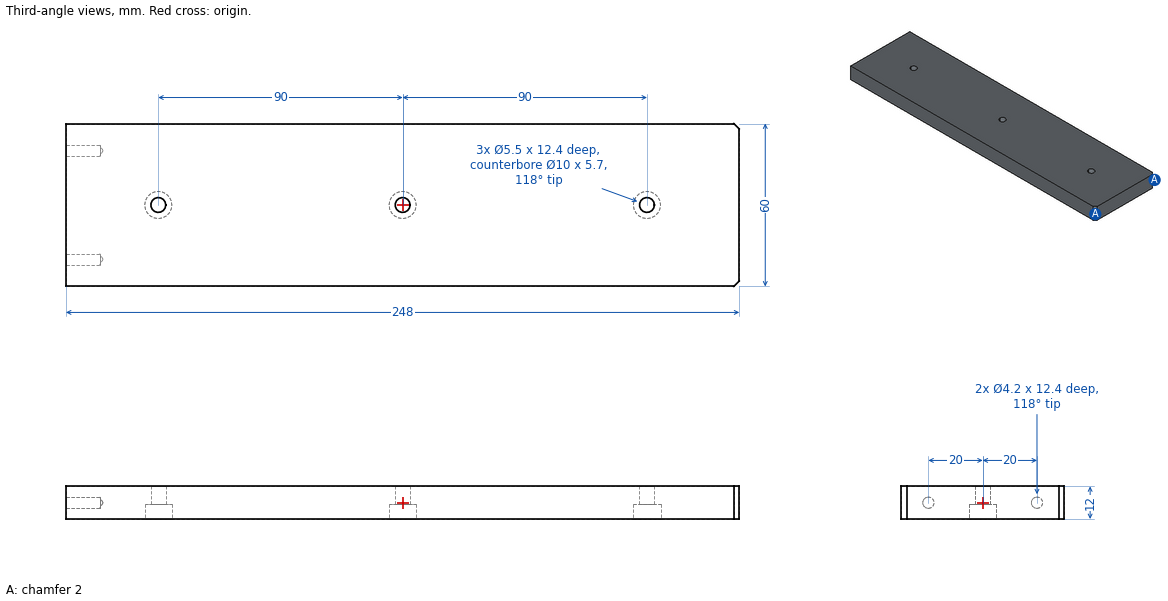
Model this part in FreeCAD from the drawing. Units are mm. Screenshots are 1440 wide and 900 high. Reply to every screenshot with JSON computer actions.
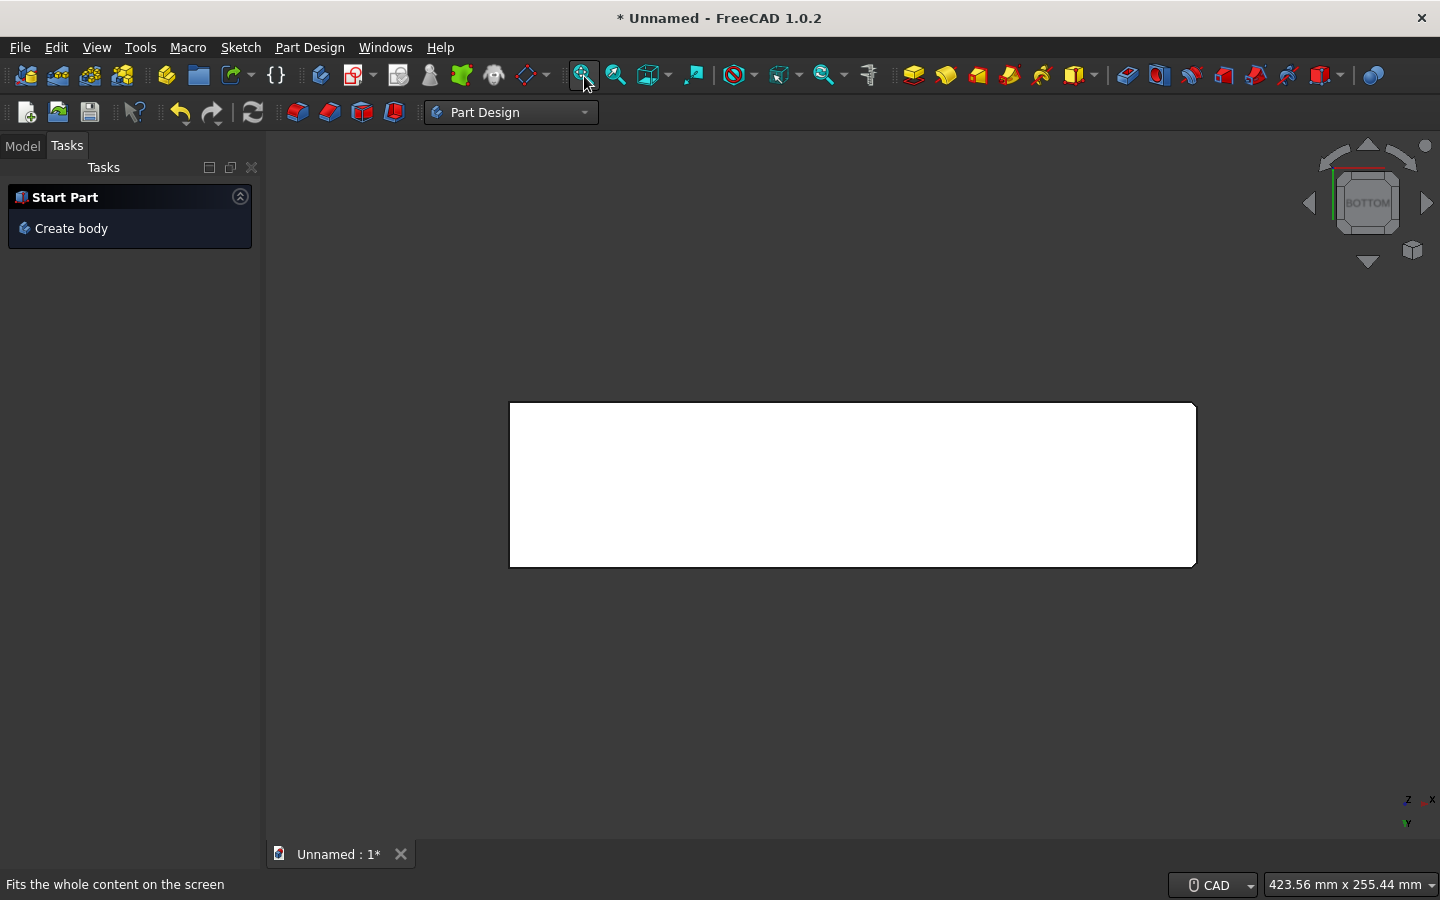
{"action": "left_click", "coordinate": [1049, 484]}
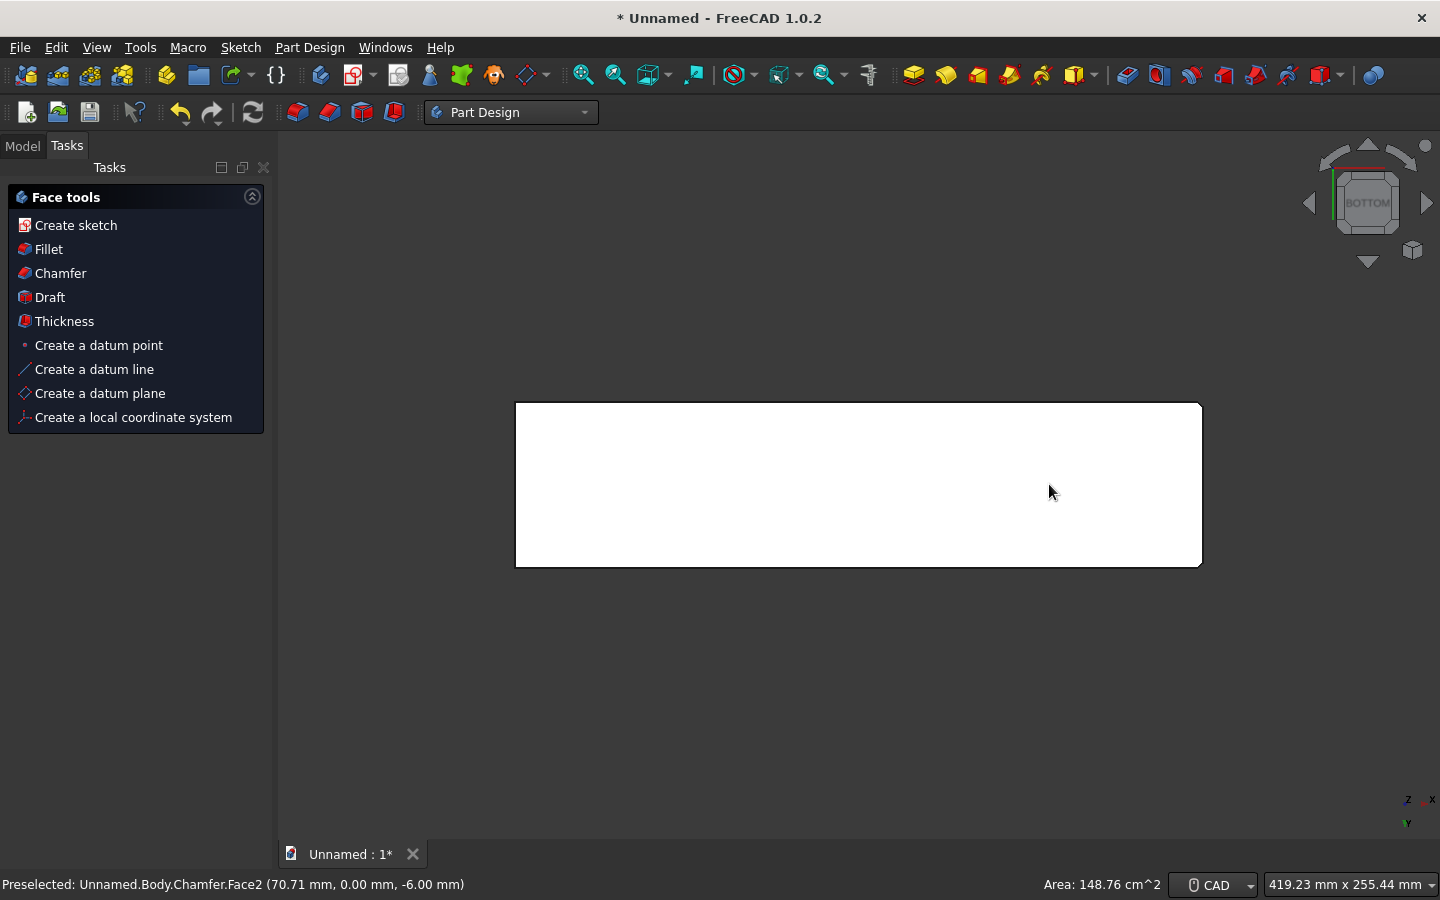
{"action": "left_click", "coordinate": [354, 76]}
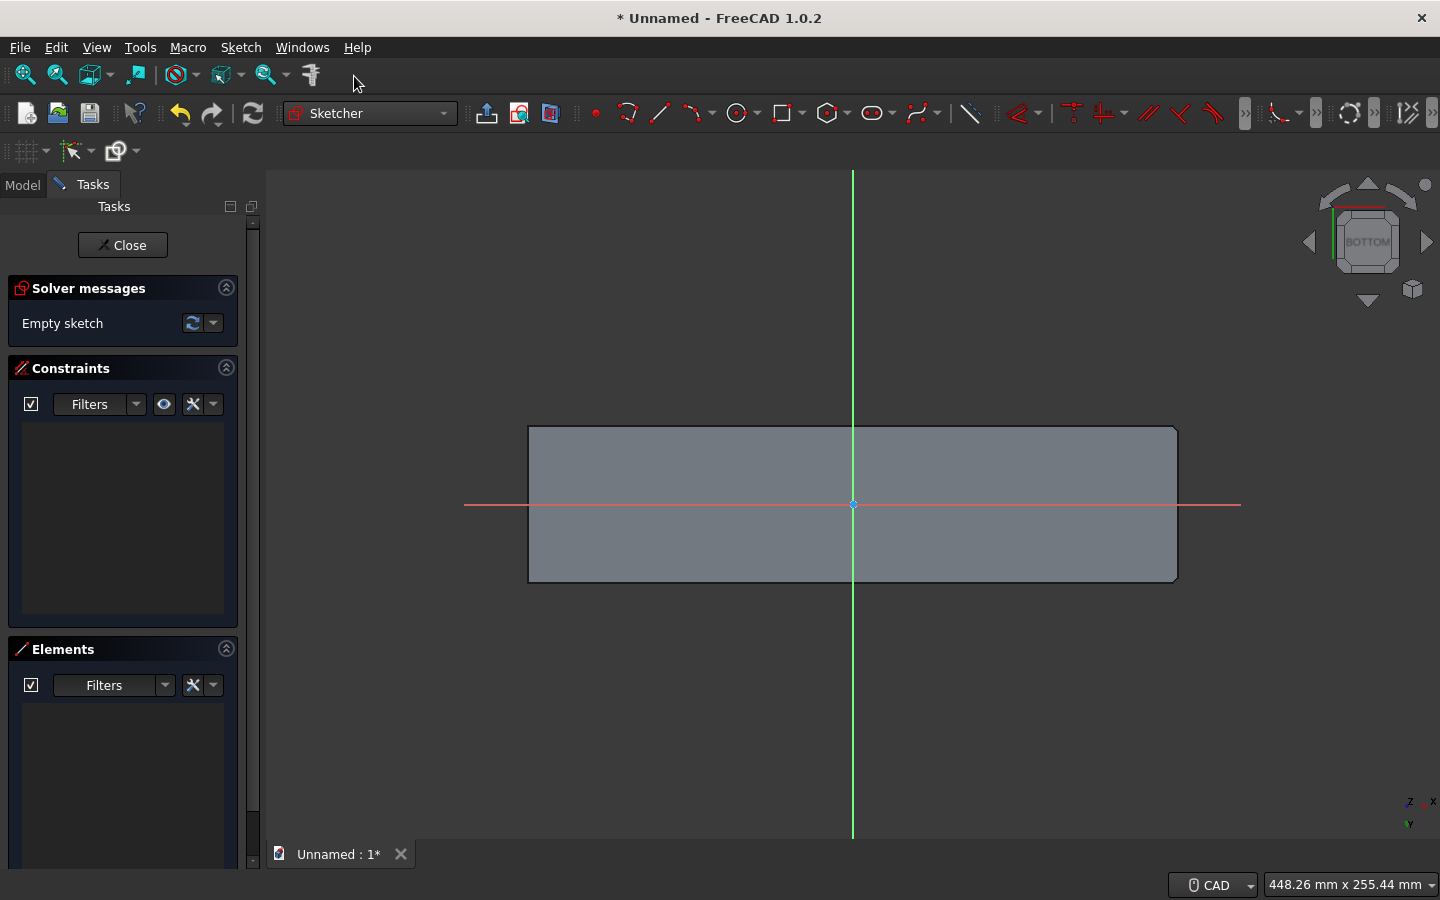
{"action": "scroll", "coordinate": [992, 504], "scroll_direction": "up", "scroll_amount": 2}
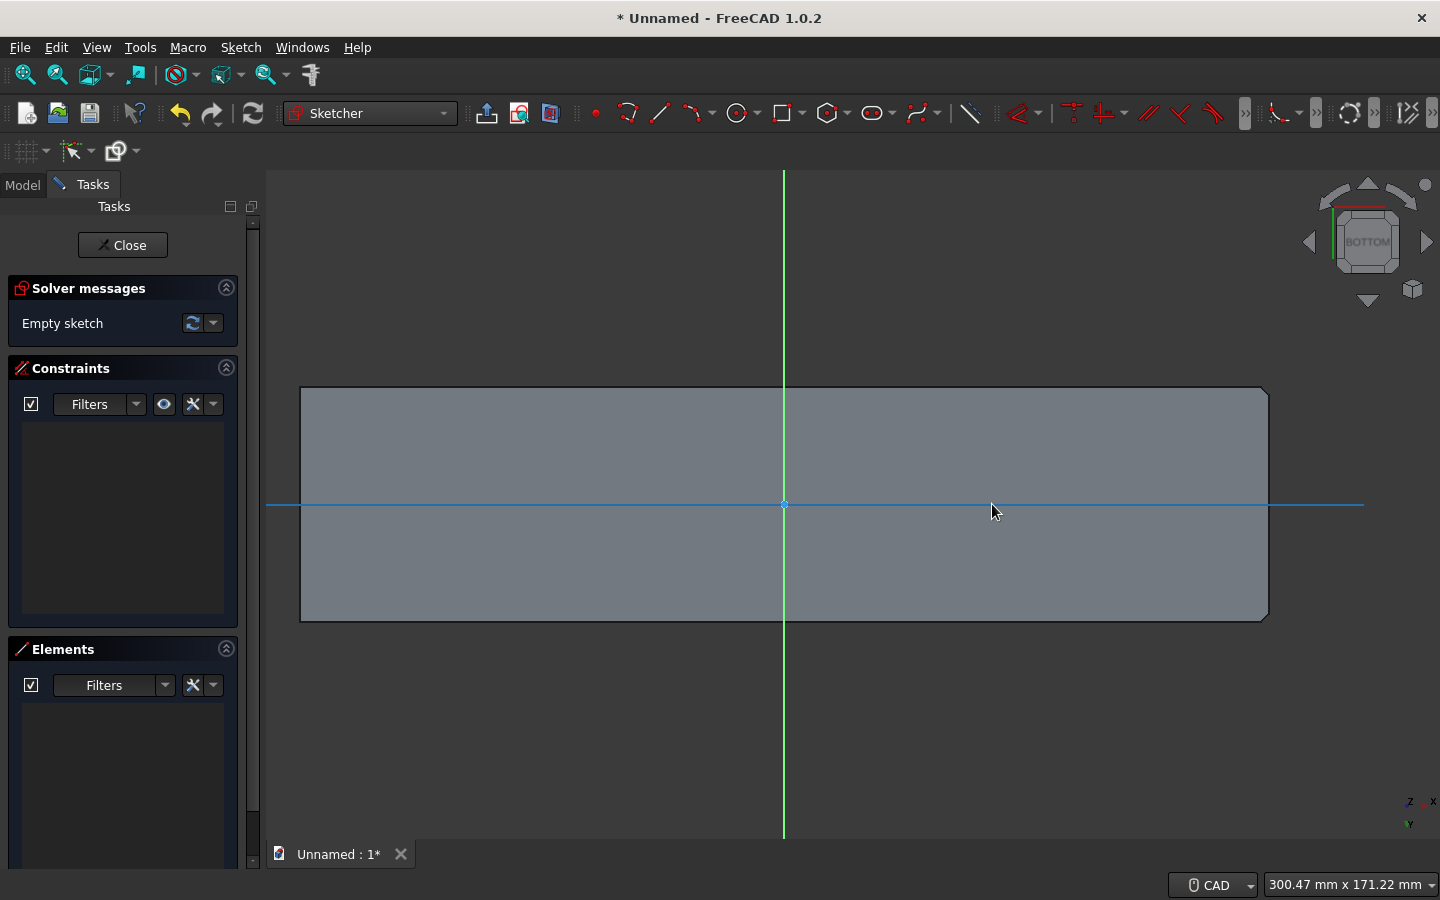
{"action": "left_click", "coordinate": [738, 114]}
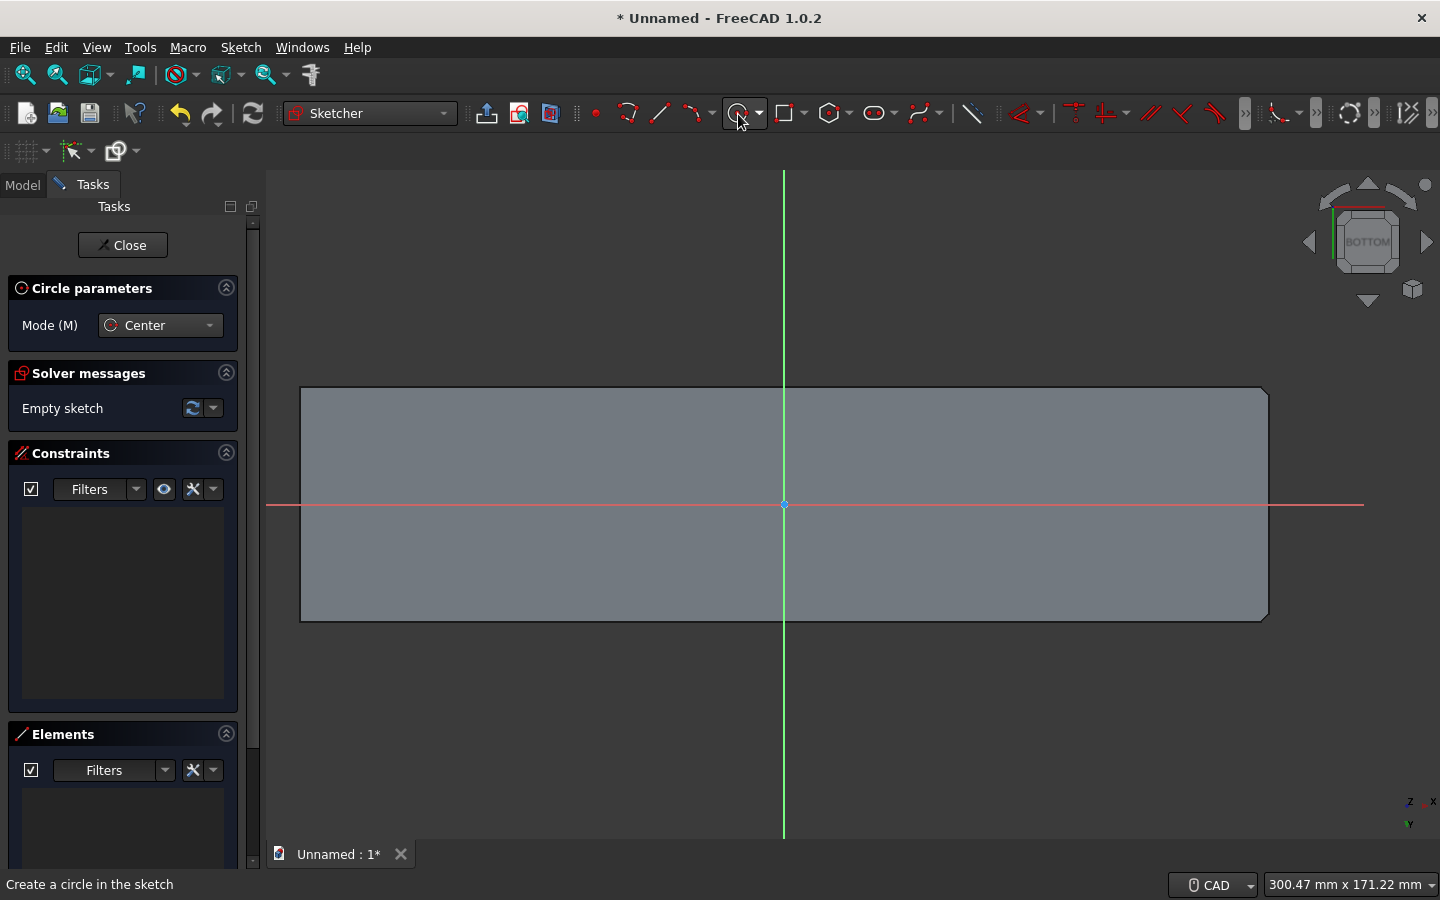
{"action": "scroll", "coordinate": [1136, 504], "scroll_direction": "up", "scroll_amount": 4}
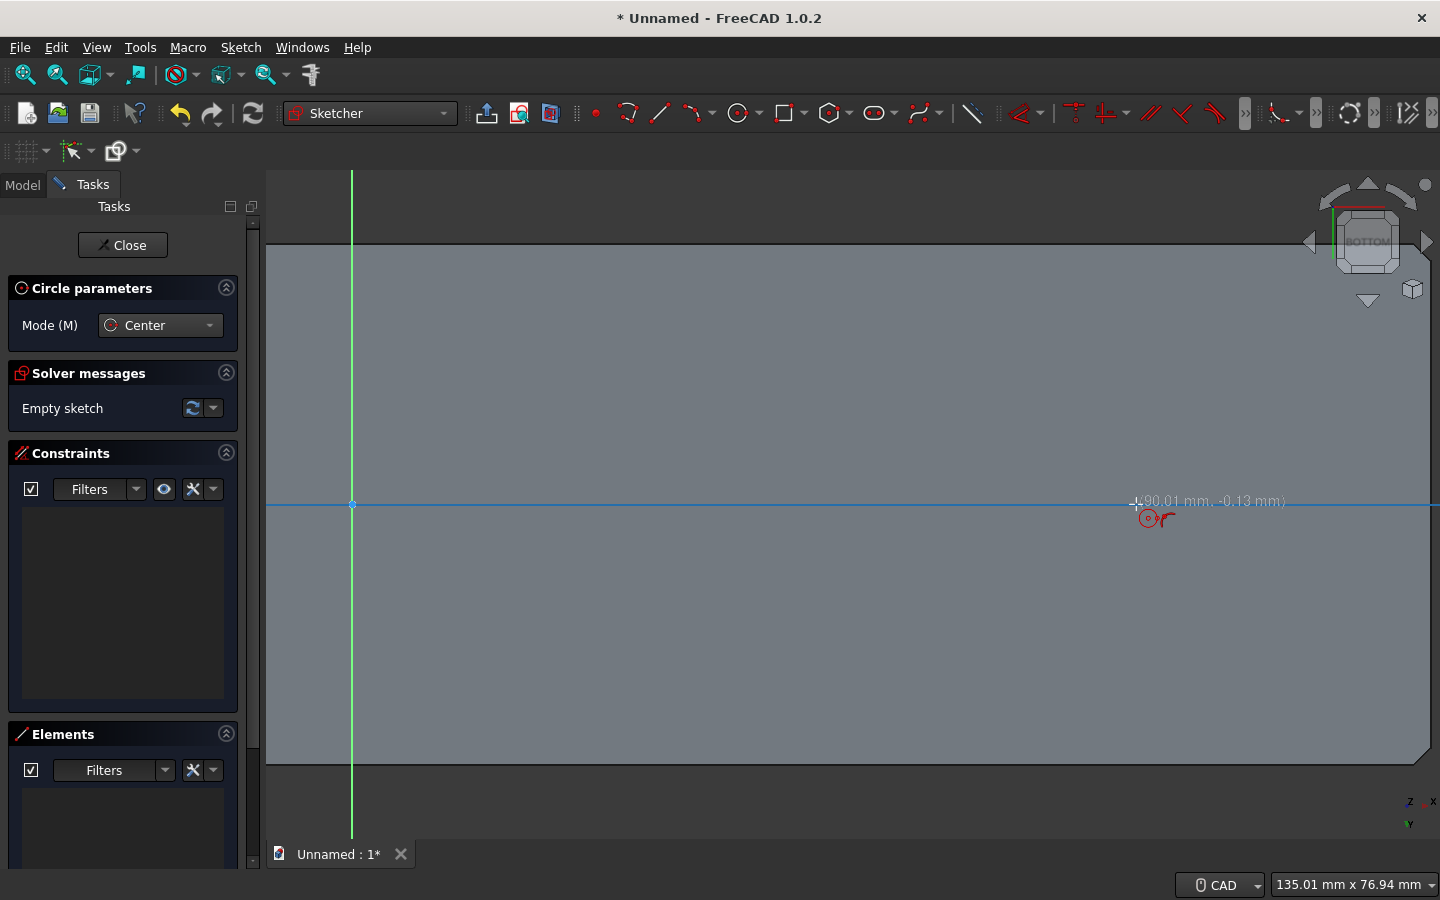
{"action": "left_click", "coordinate": [1135, 504]}
{"action": "left_click", "coordinate": [1152, 488]}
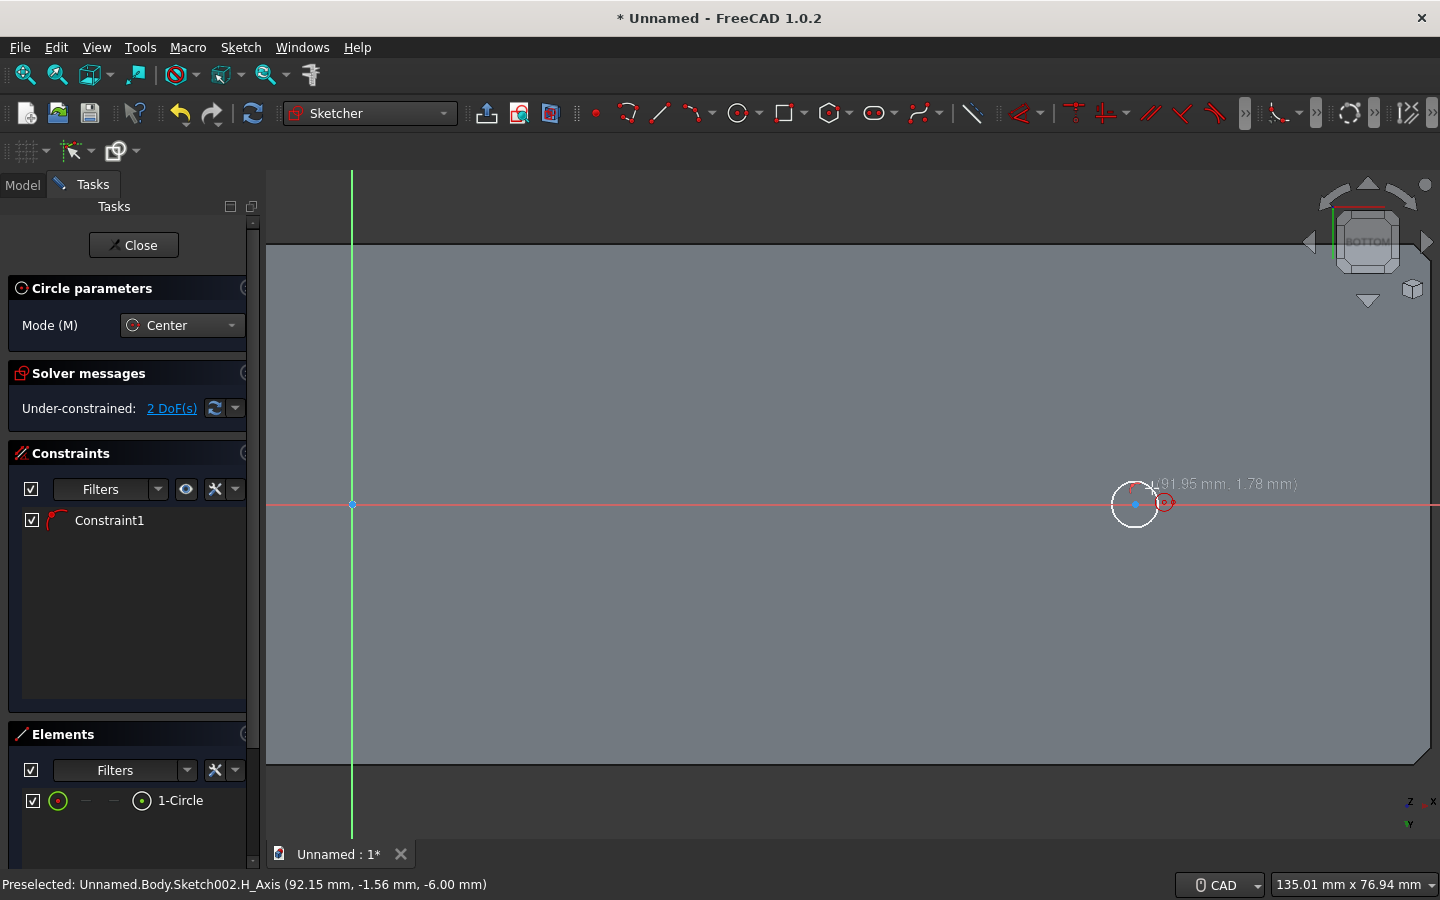
{"action": "left_click", "coordinate": [352, 504]}
{"action": "left_click", "coordinate": [369, 488]}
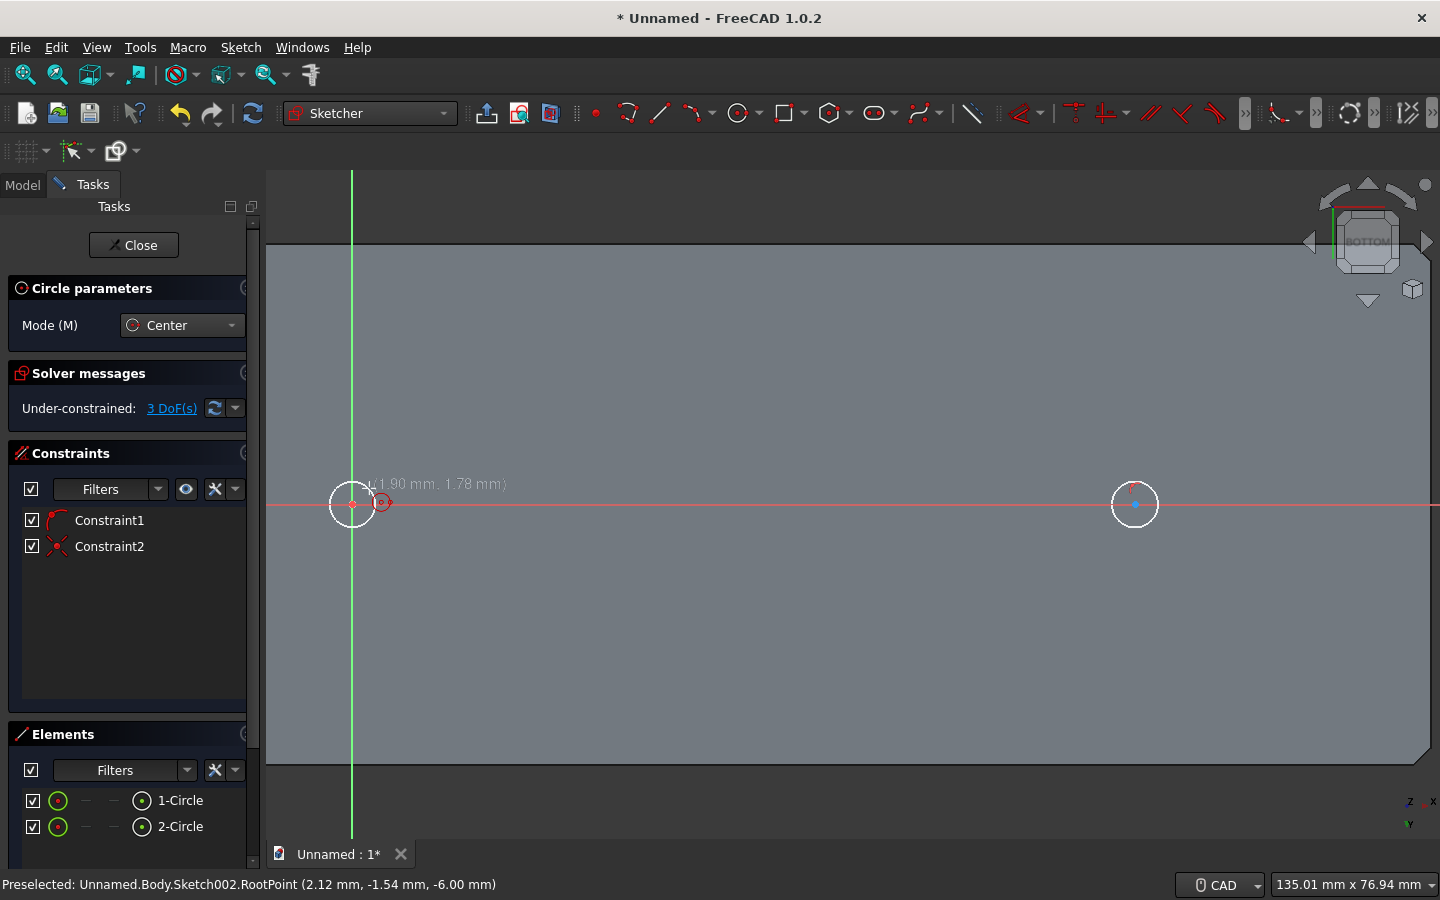
{"action": "scroll", "coordinate": [1137, 505], "scroll_direction": "down", "scroll_amount": 4}